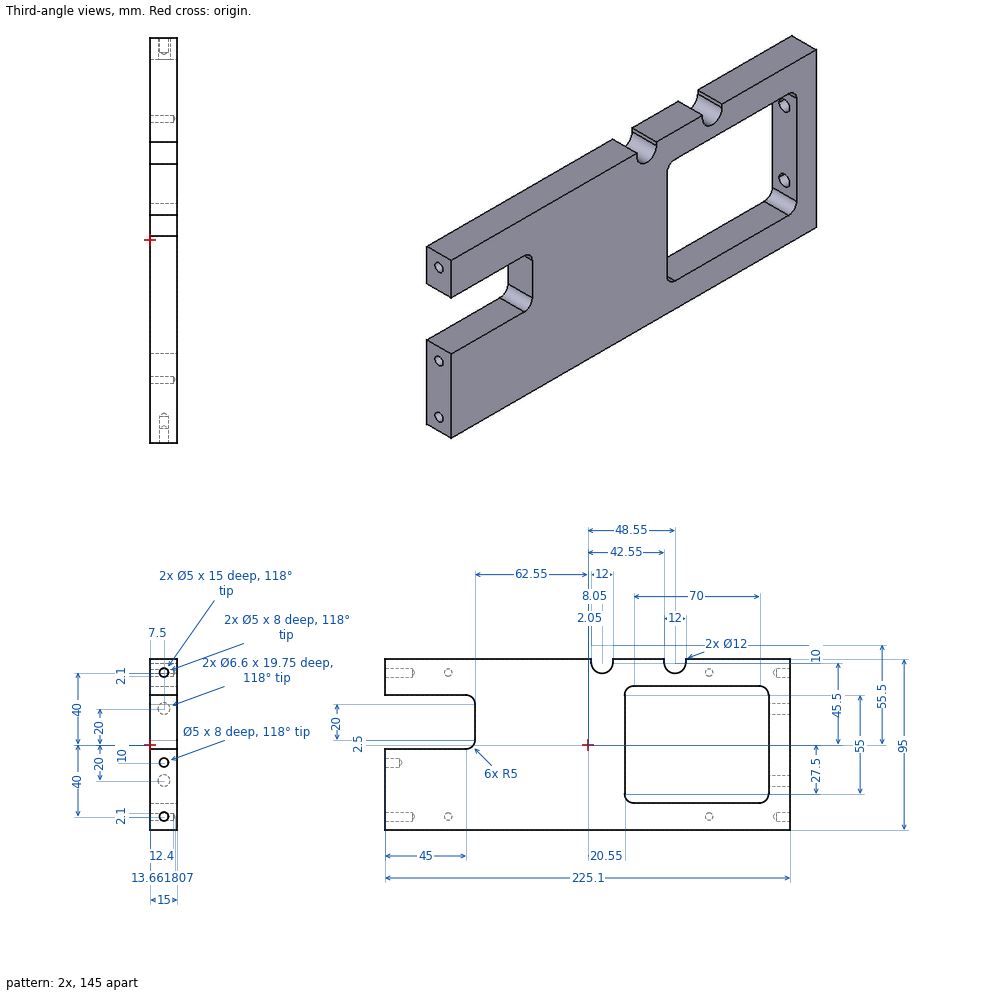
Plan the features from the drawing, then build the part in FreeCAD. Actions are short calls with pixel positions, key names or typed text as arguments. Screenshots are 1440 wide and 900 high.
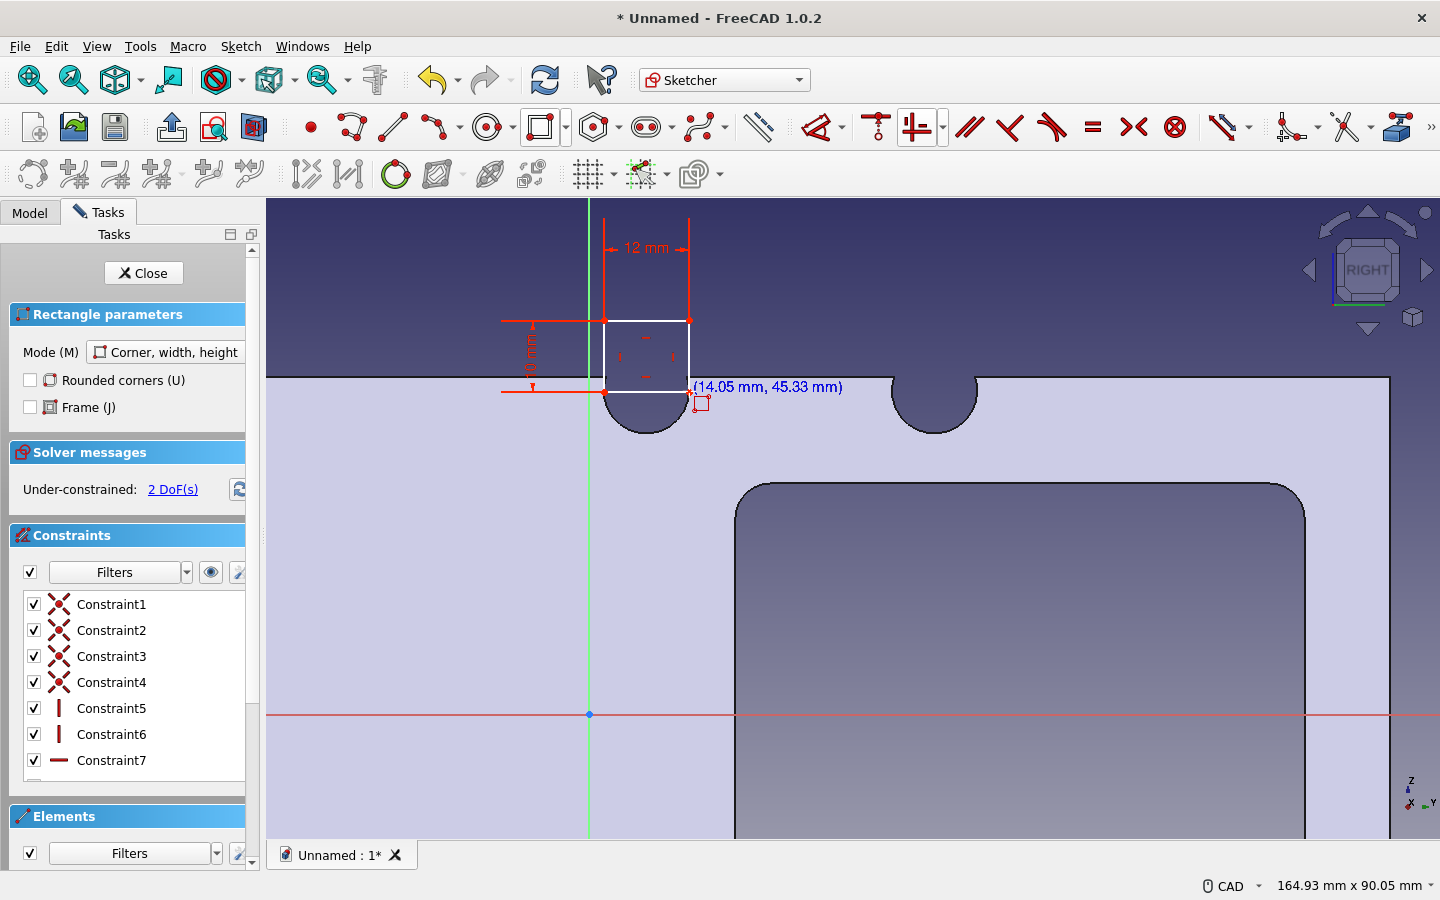
click(892, 320)
move(977, 391)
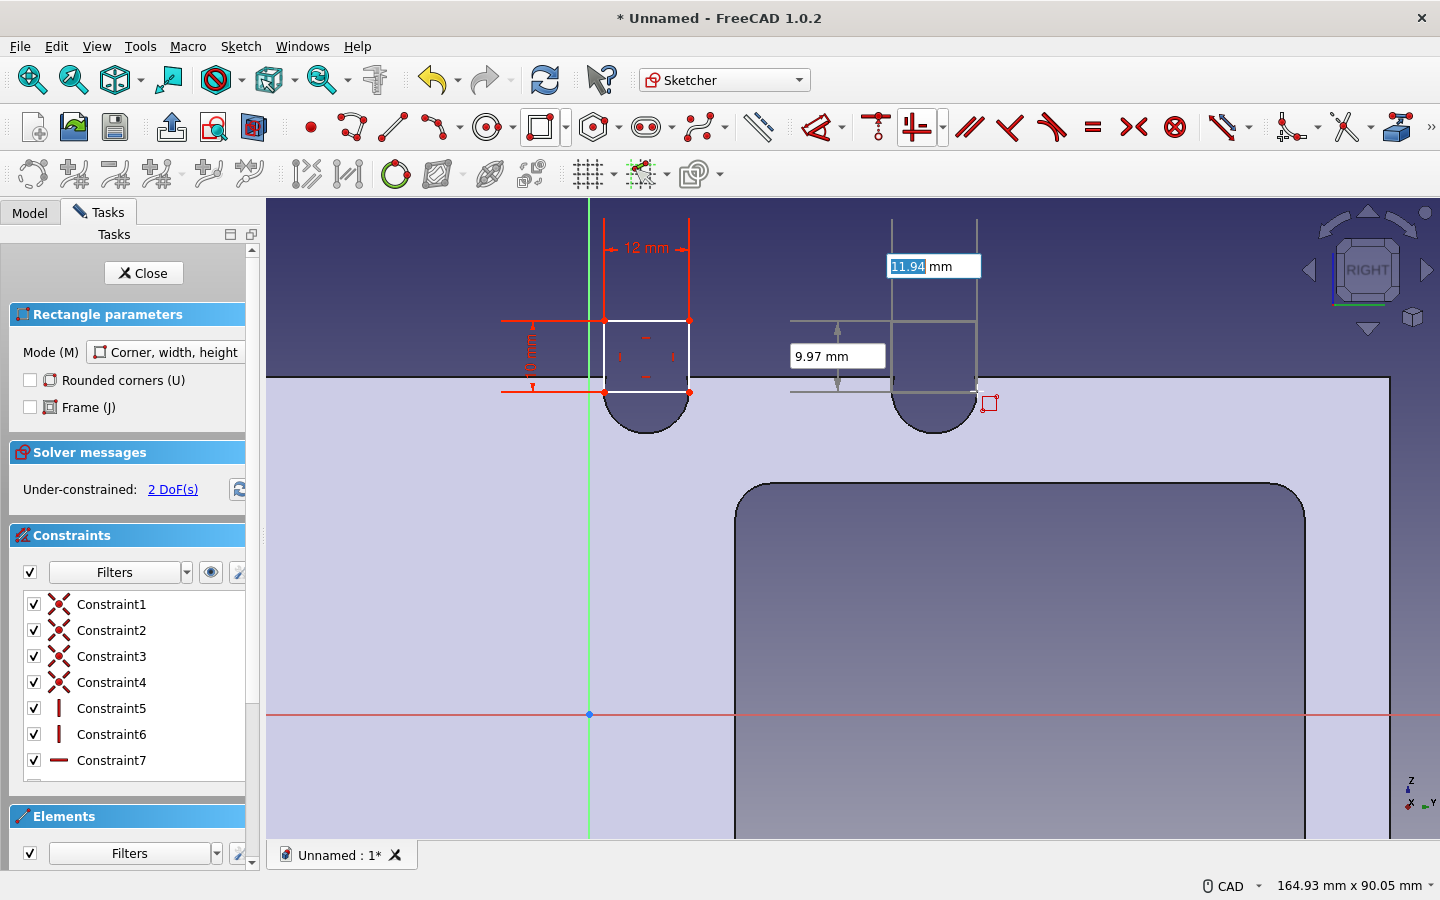
text(12)
key(Tab)
text(10)
key(Return)
key(Escape)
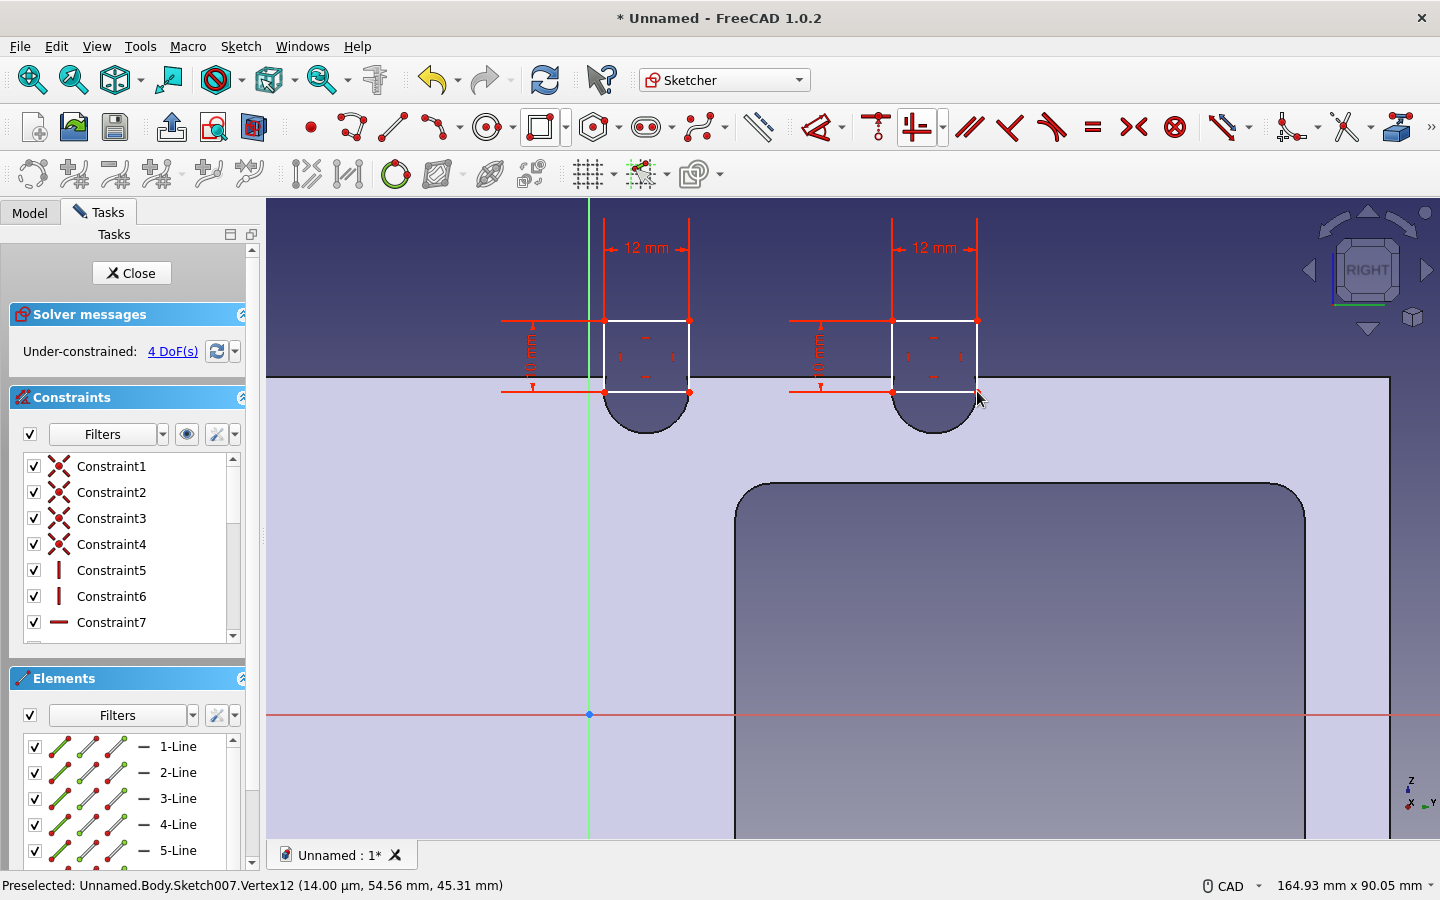
click(816, 128)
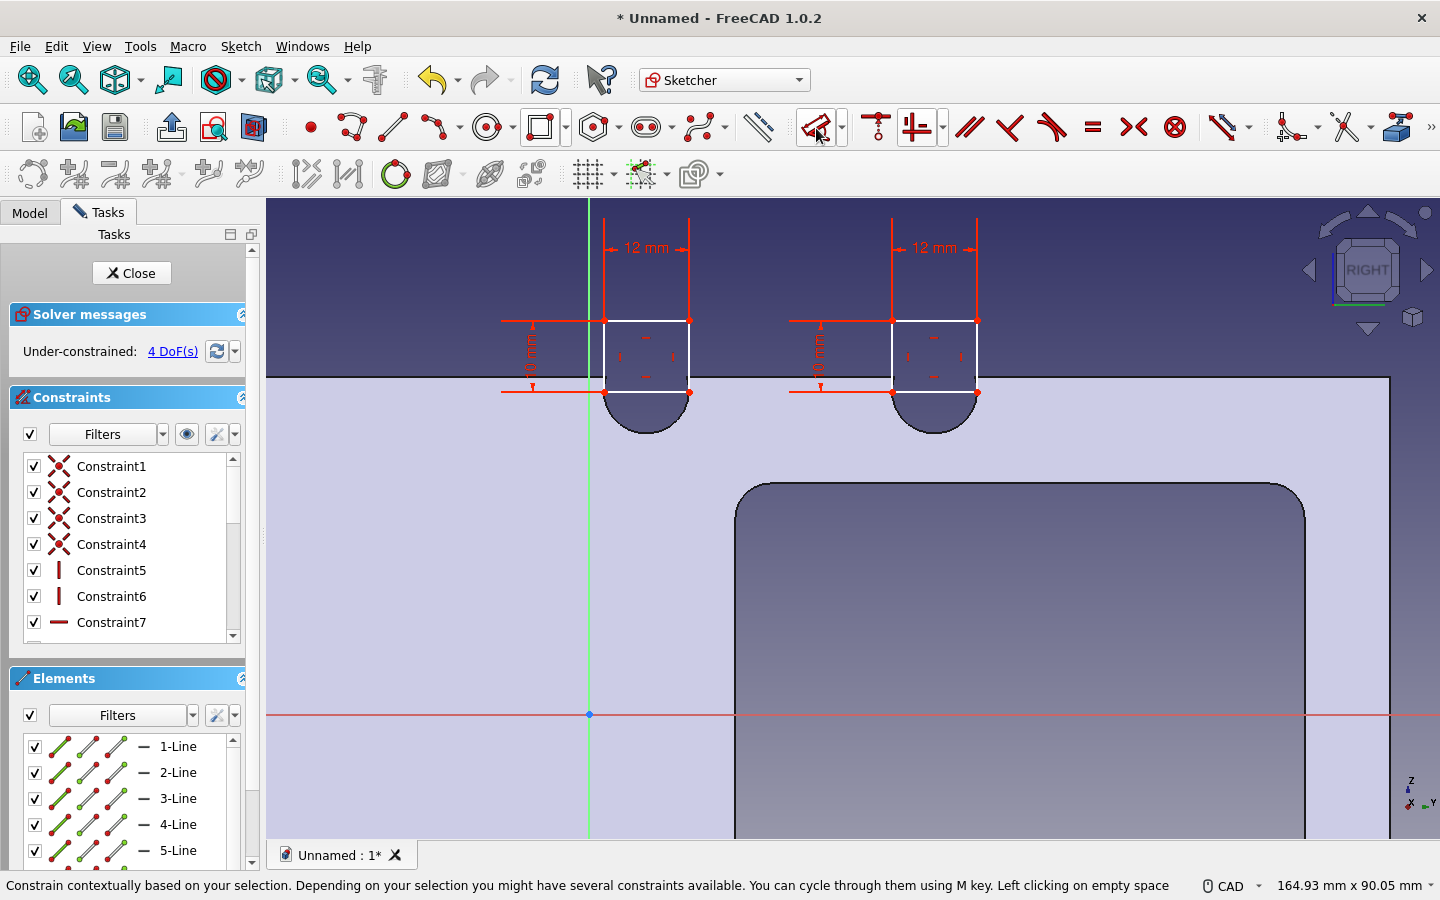
scroll(604, 321, up, 6)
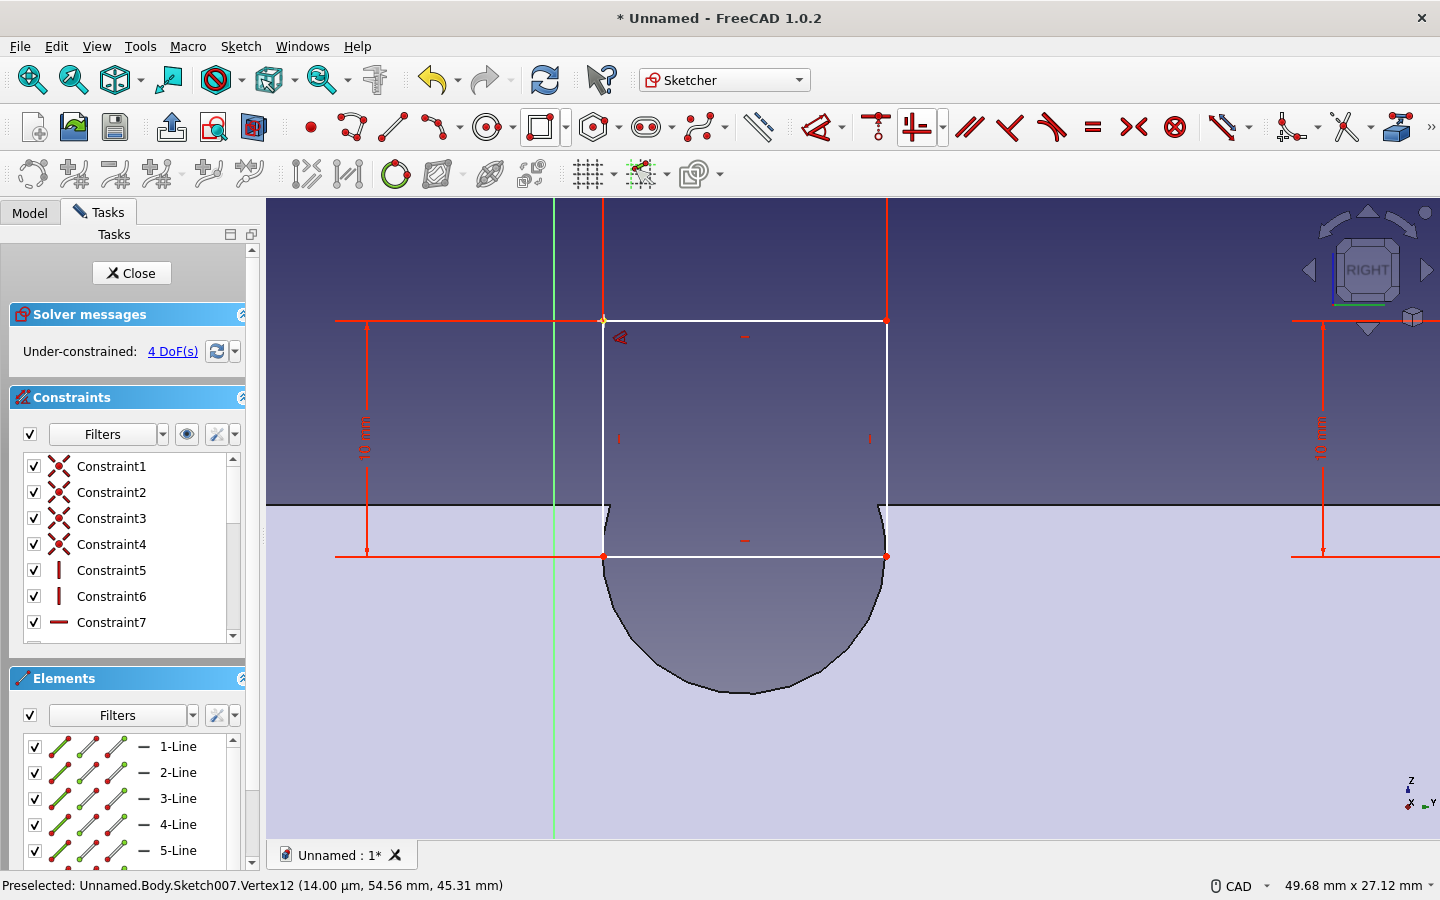
click(603, 321)
click(578, 287)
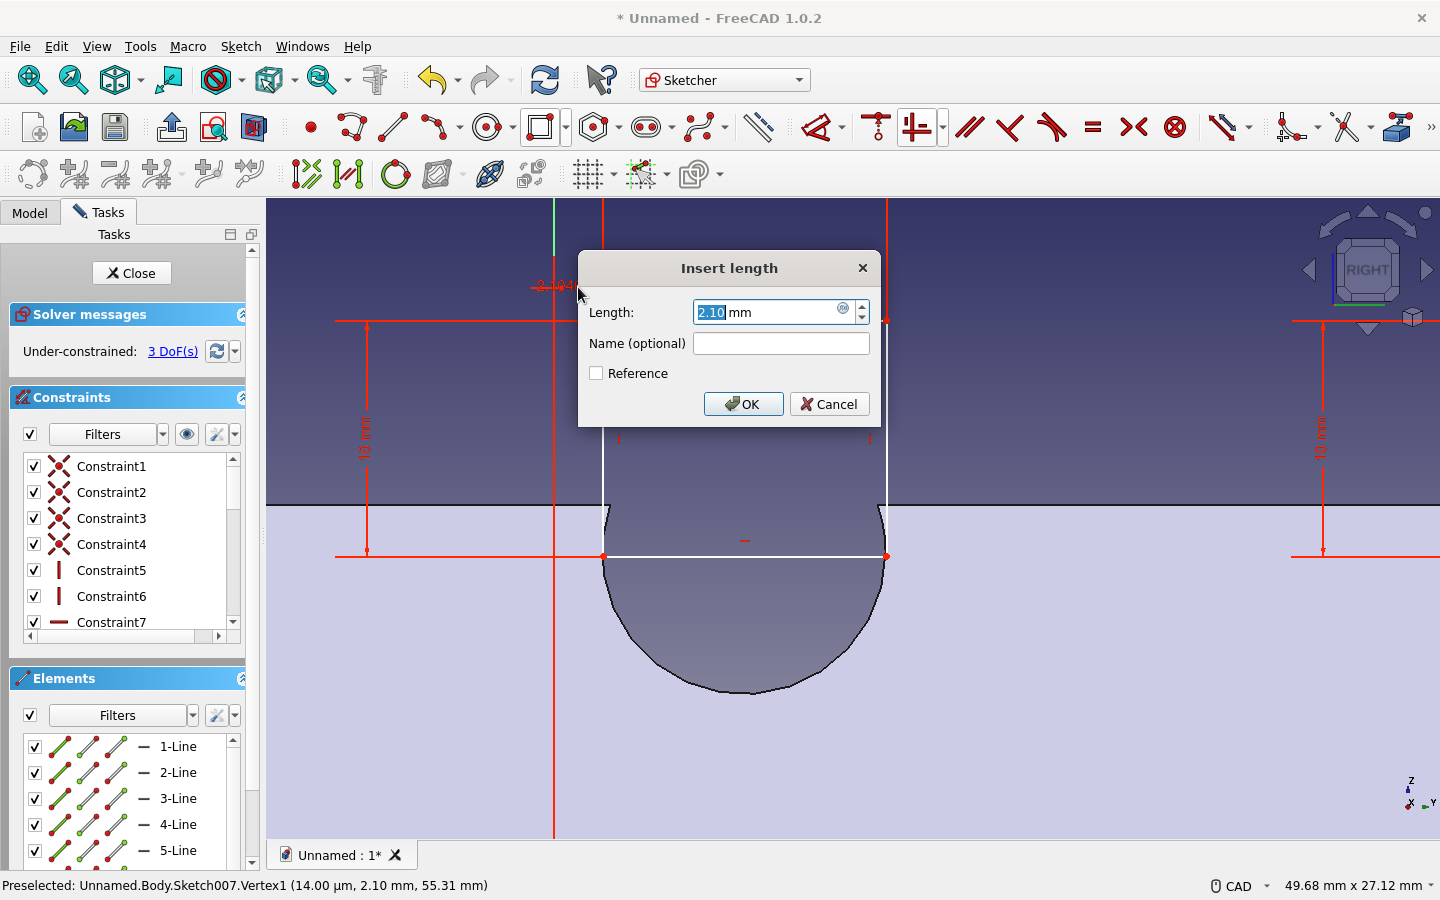
text(2.05)
key(Return)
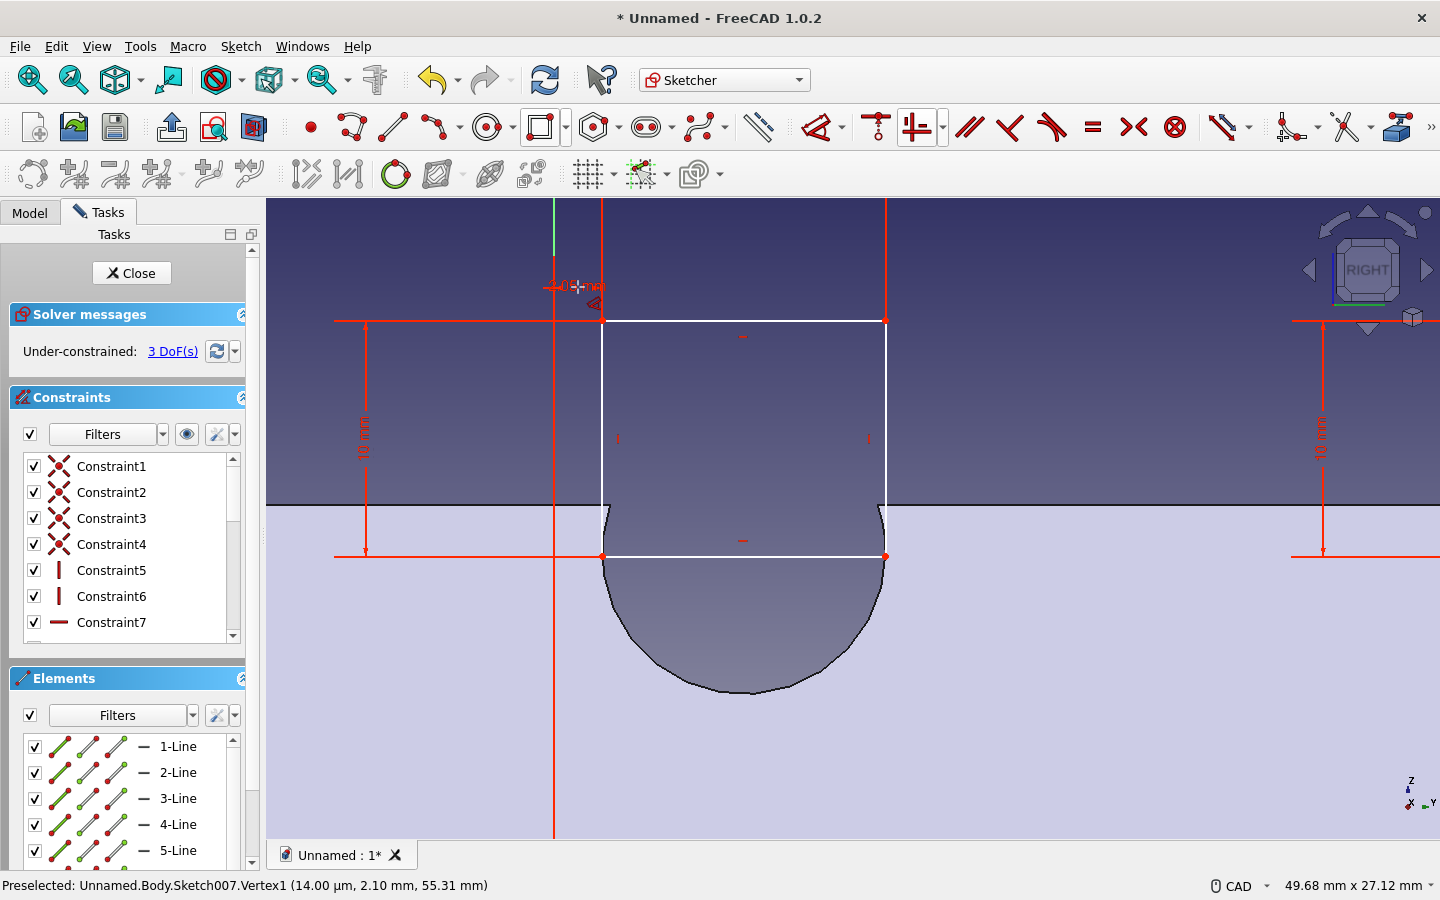
click(602, 321)
click(520, 566)